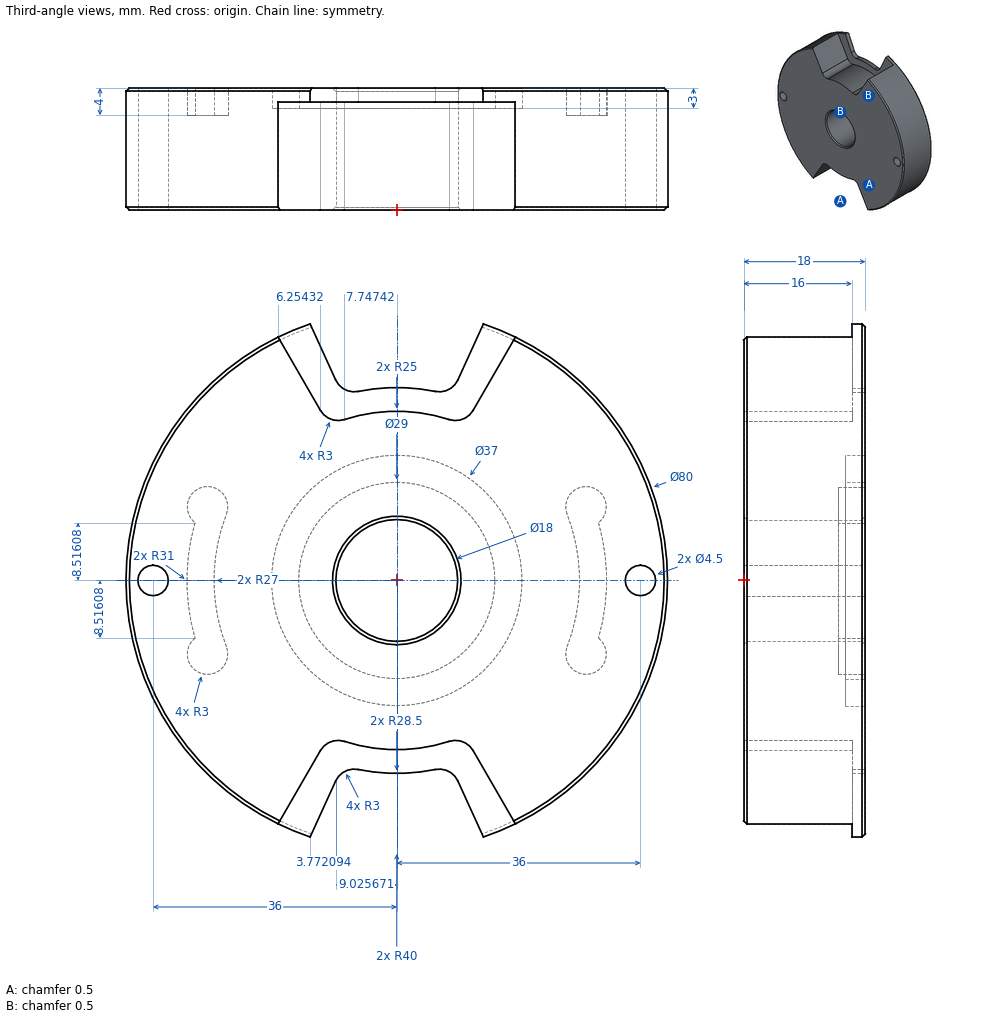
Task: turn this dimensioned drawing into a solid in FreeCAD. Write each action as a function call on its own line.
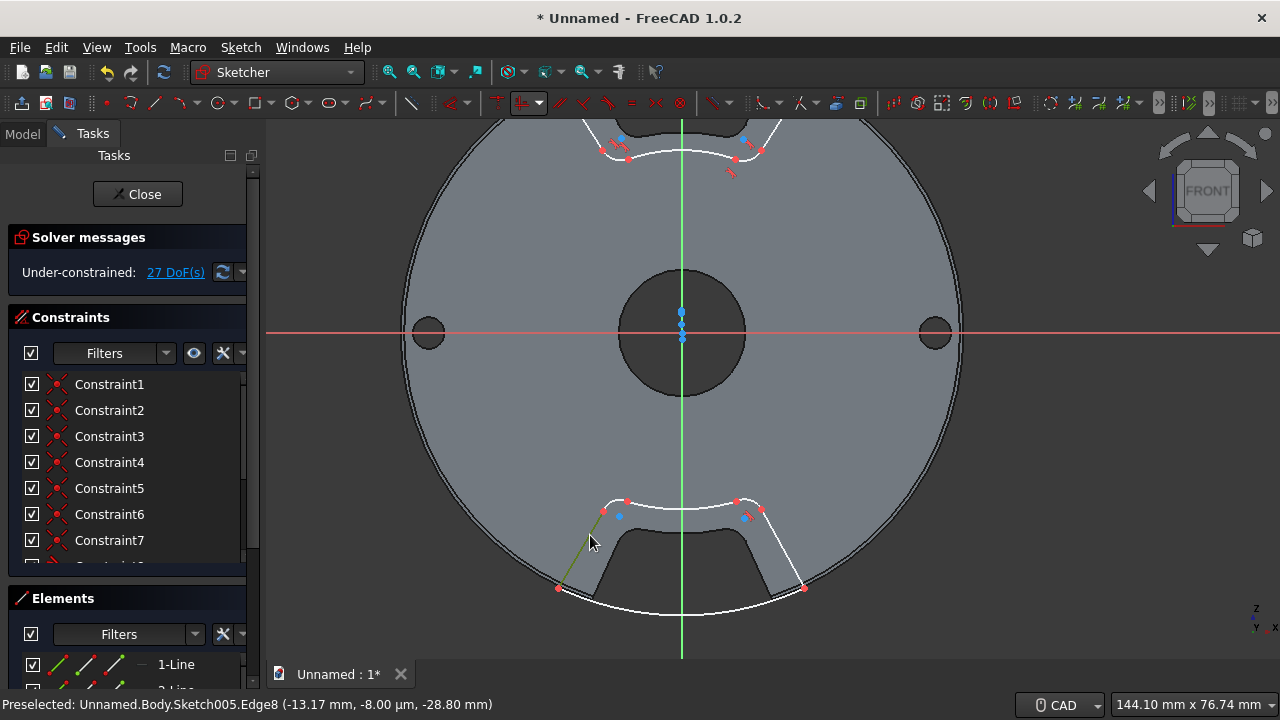
click(613, 501)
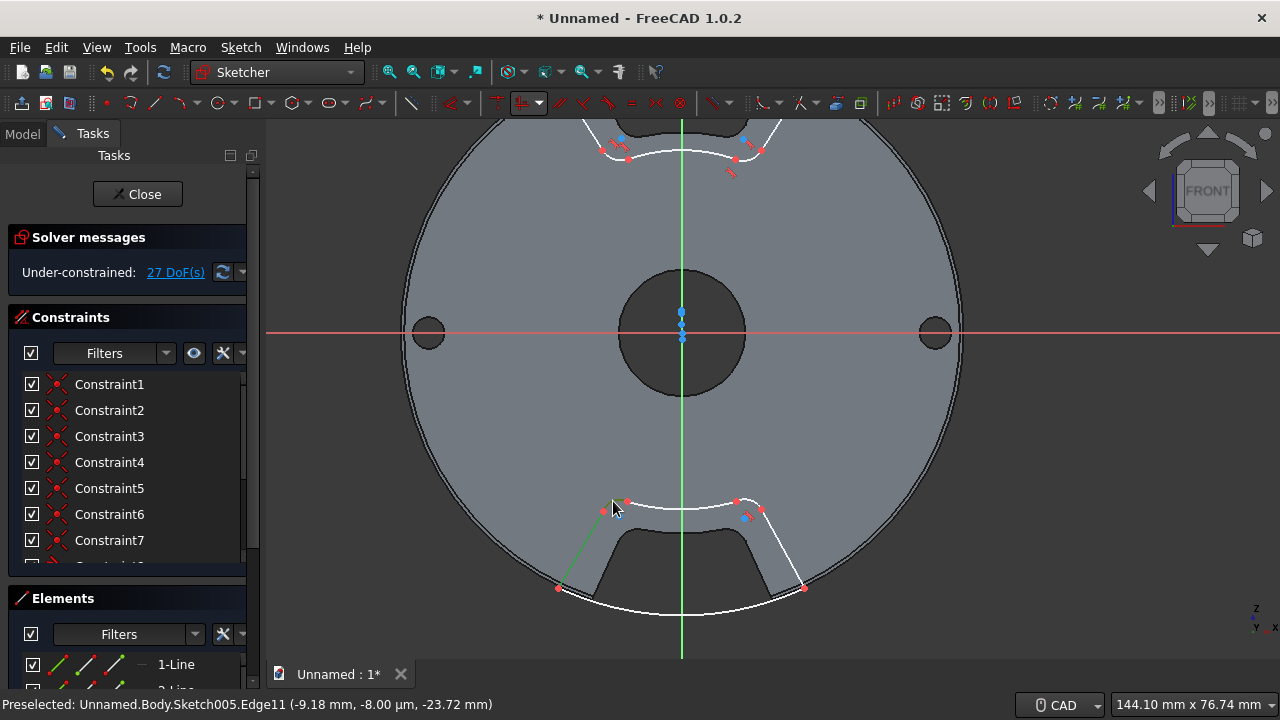
click(608, 104)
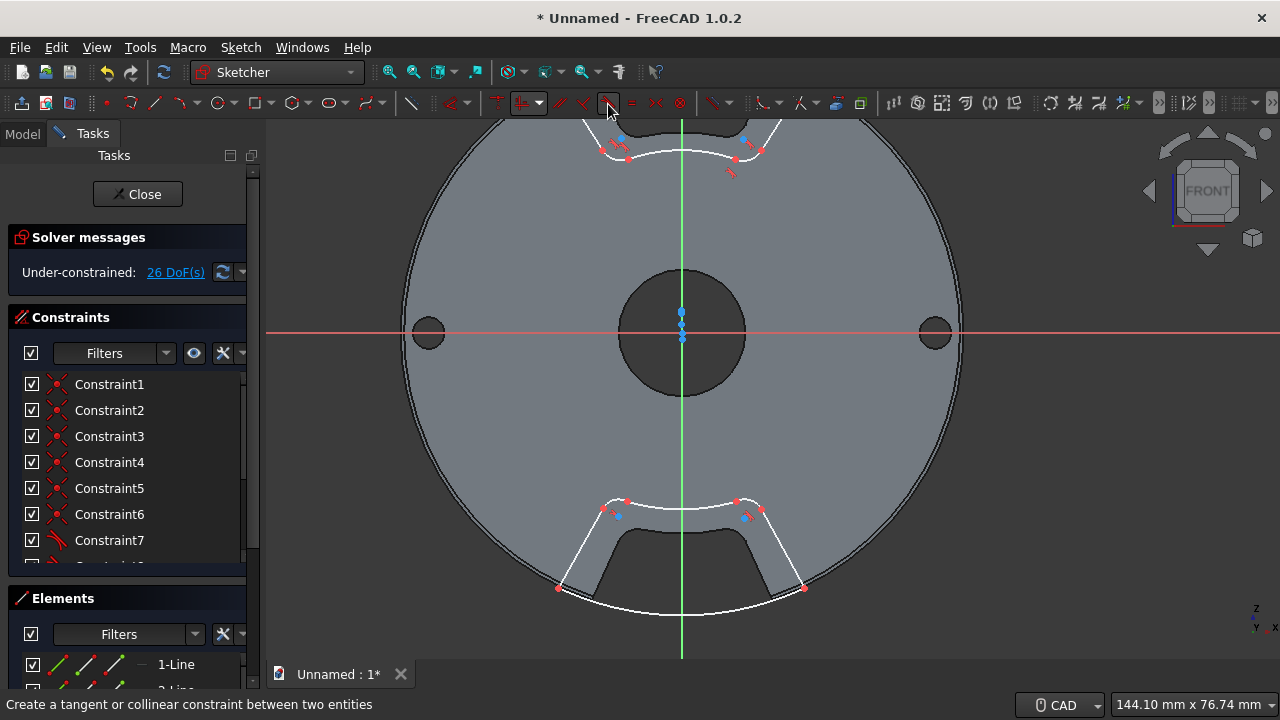
click(750, 500)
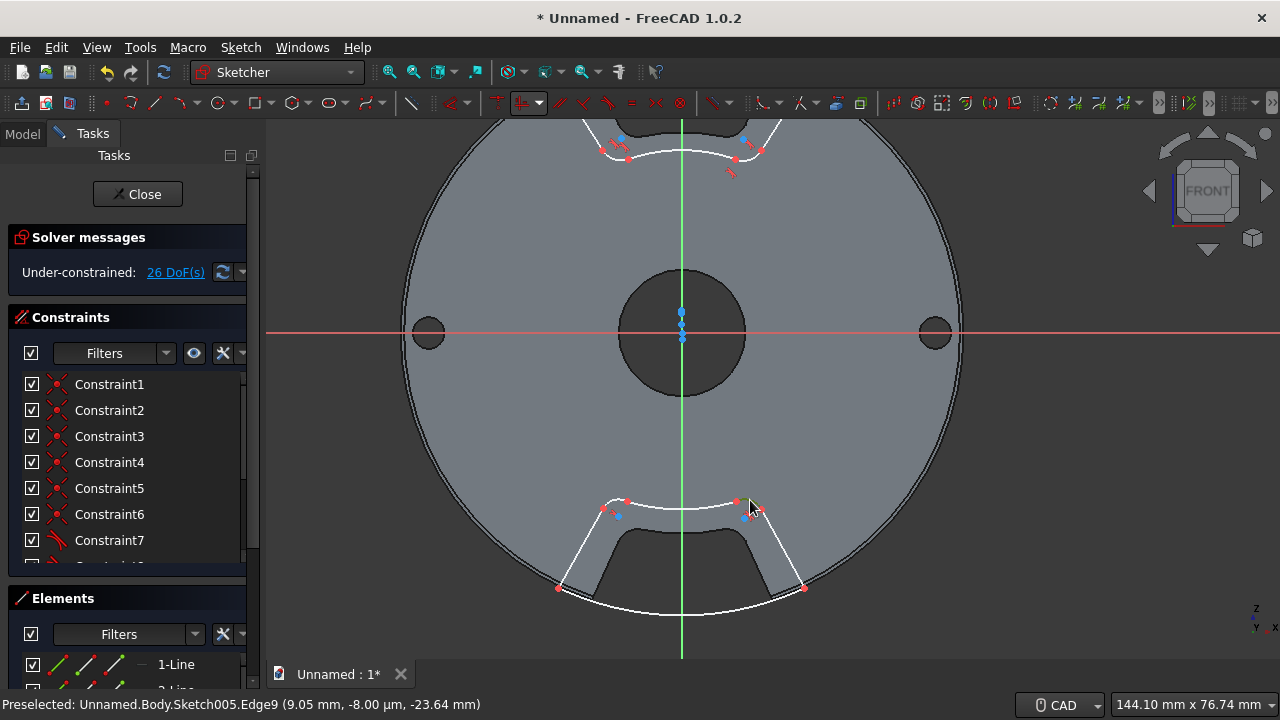
click(660, 508)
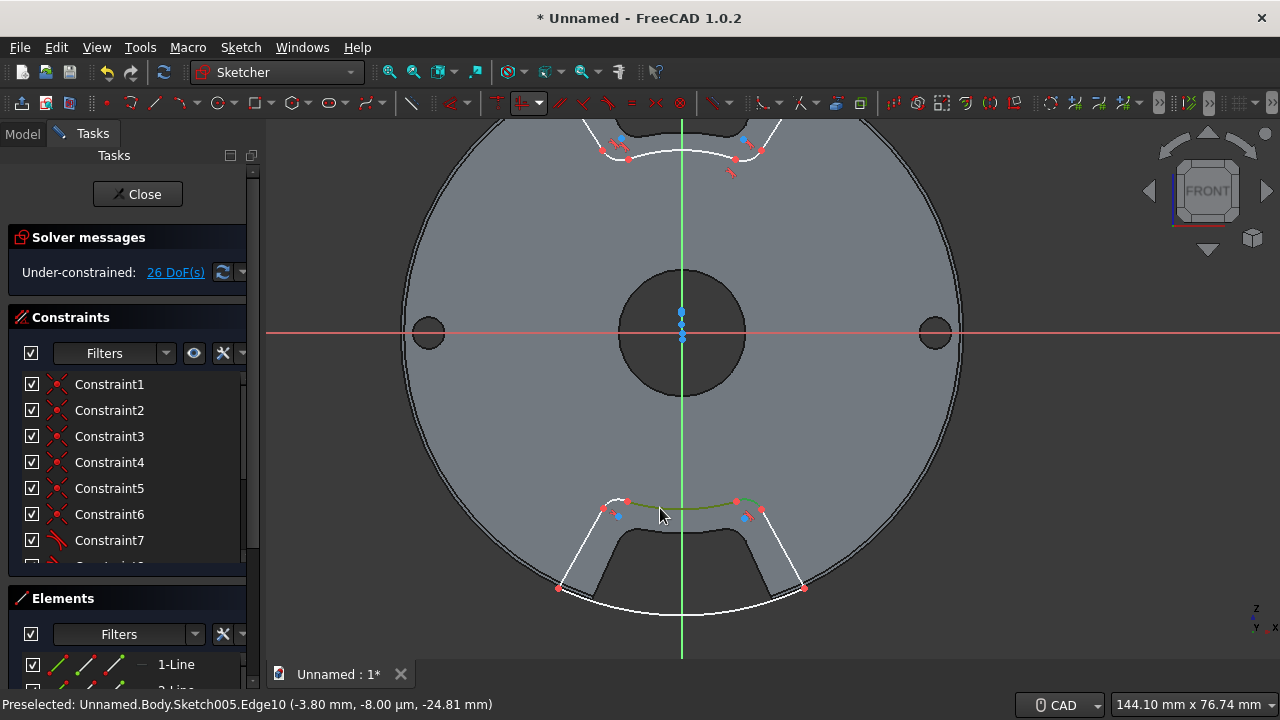
click(608, 104)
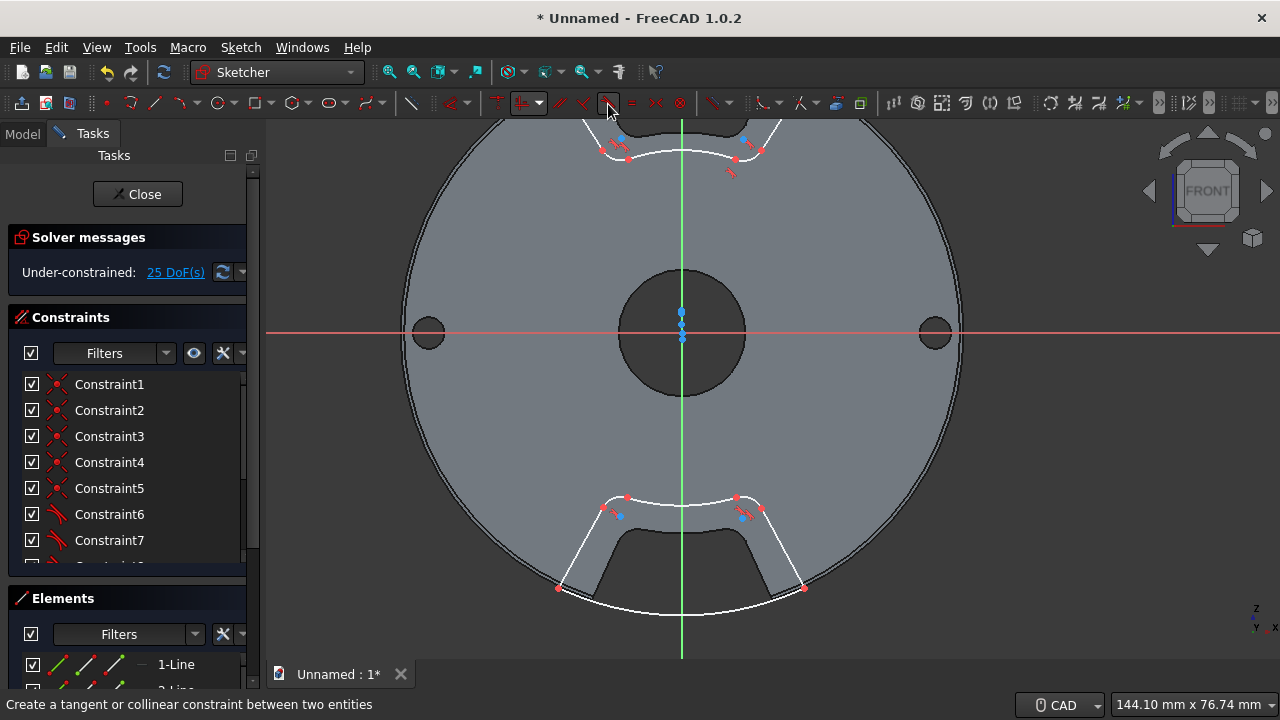
click(660, 504)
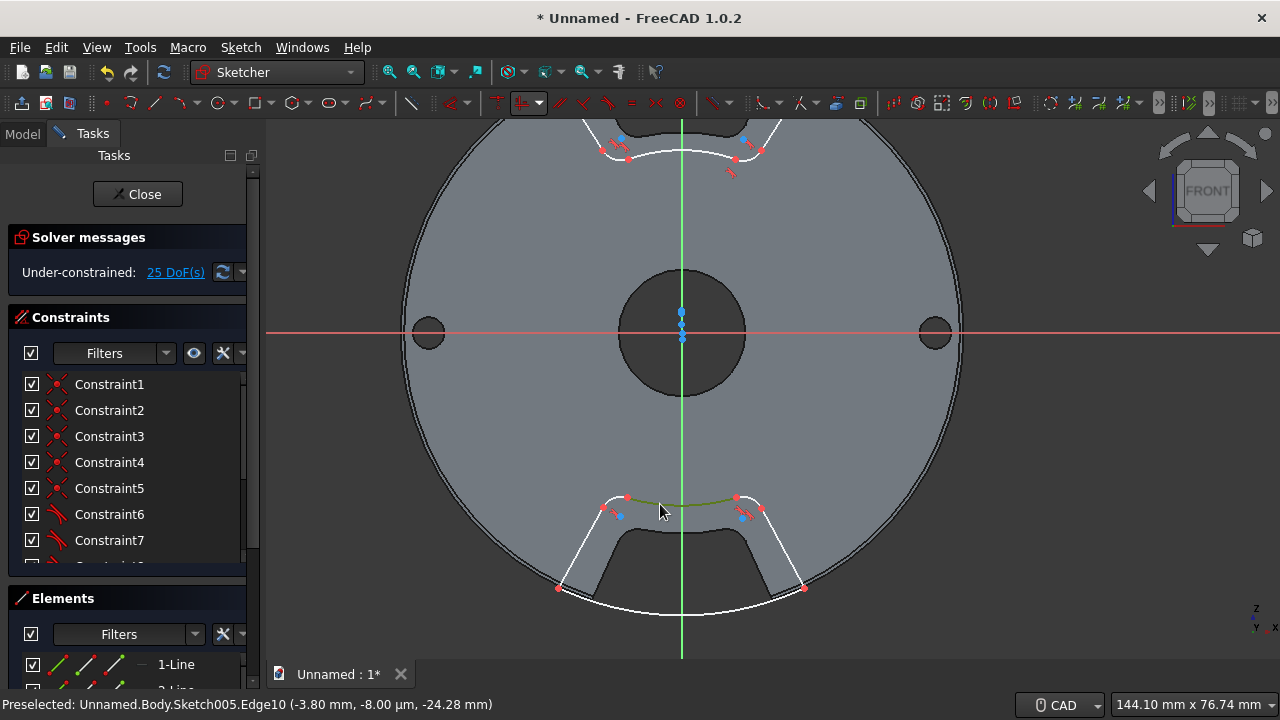
click(614, 498)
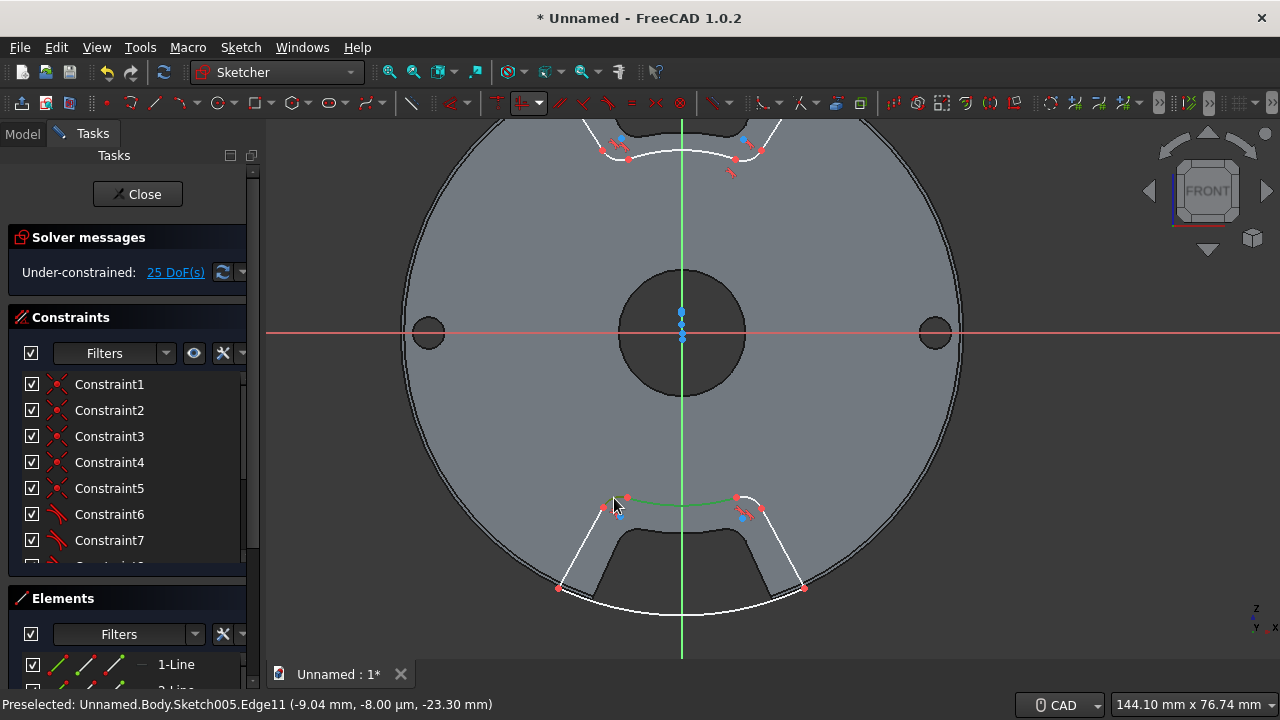
click(608, 104)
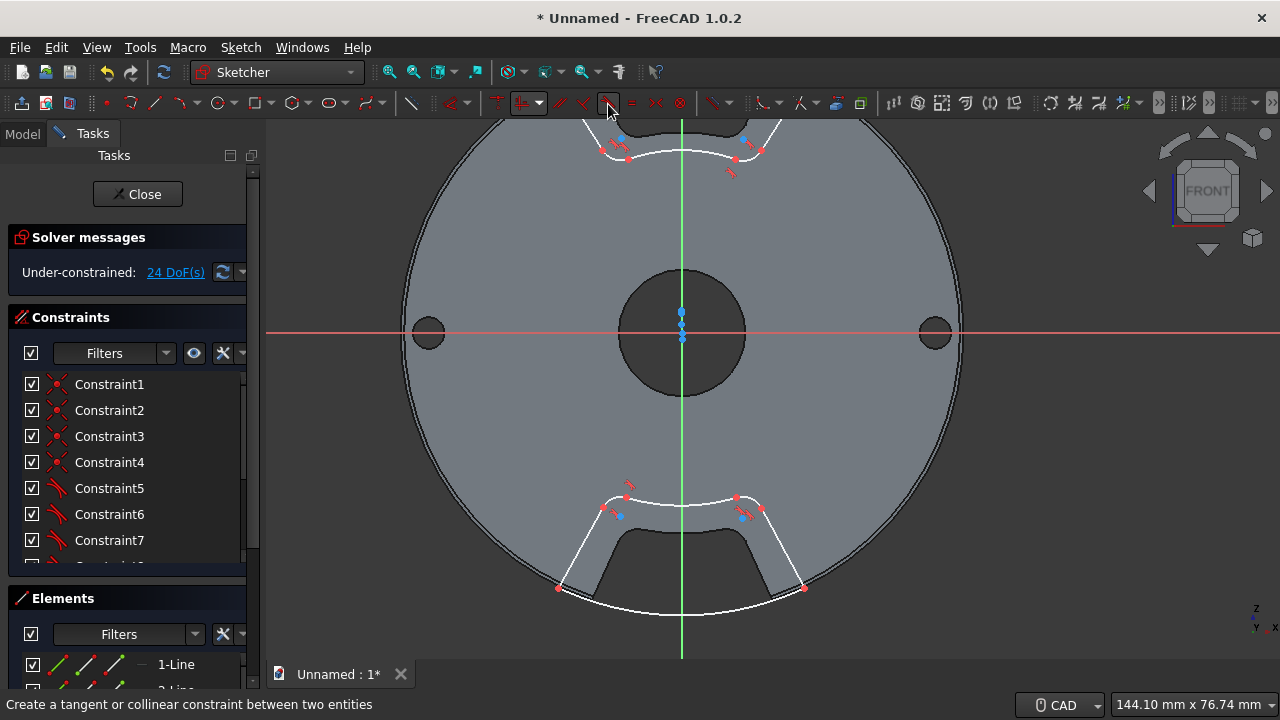
click(704, 152)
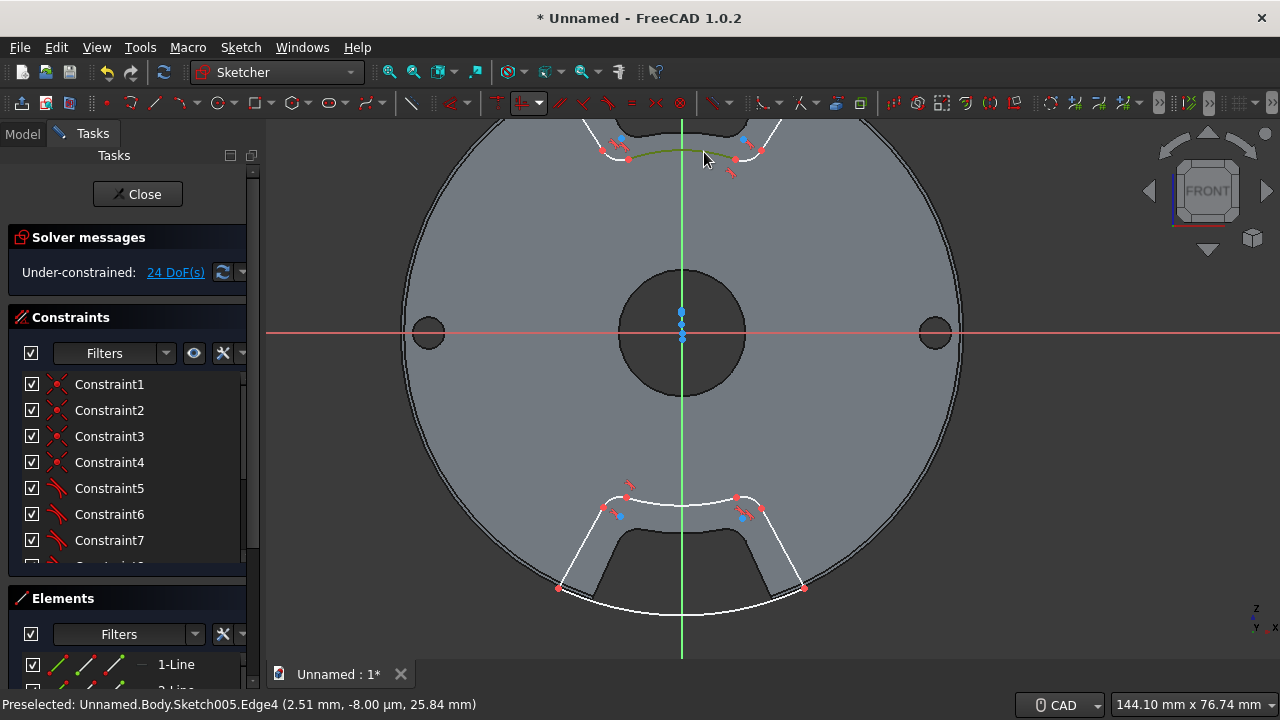
scroll(750, 503, down, 2)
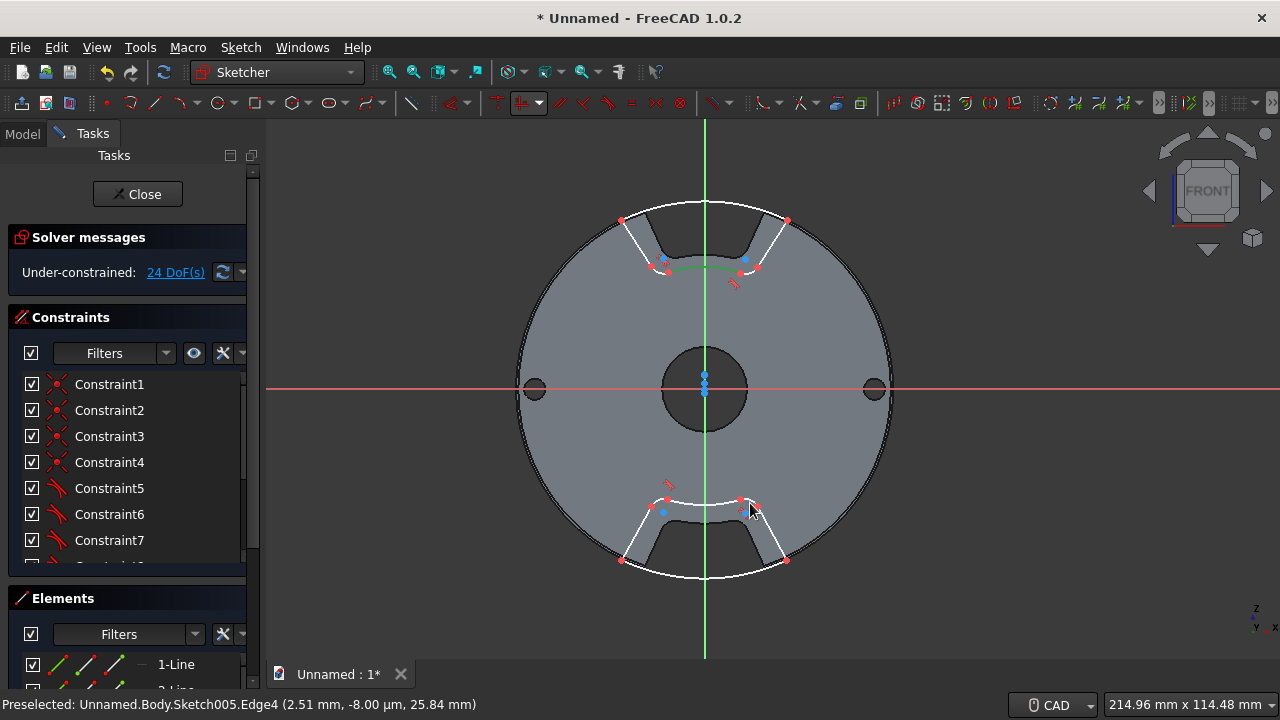
click(739, 205)